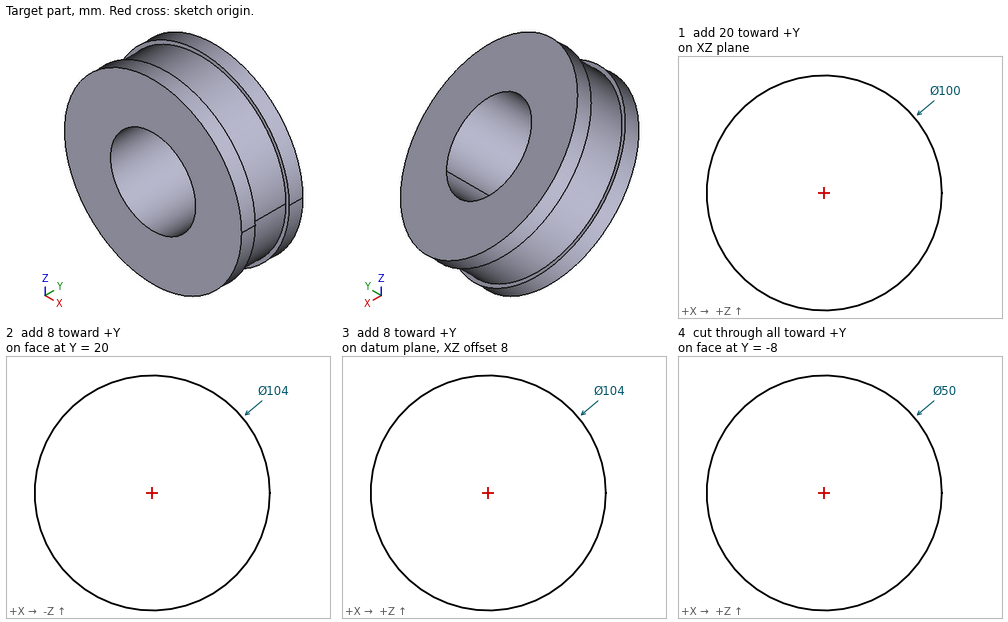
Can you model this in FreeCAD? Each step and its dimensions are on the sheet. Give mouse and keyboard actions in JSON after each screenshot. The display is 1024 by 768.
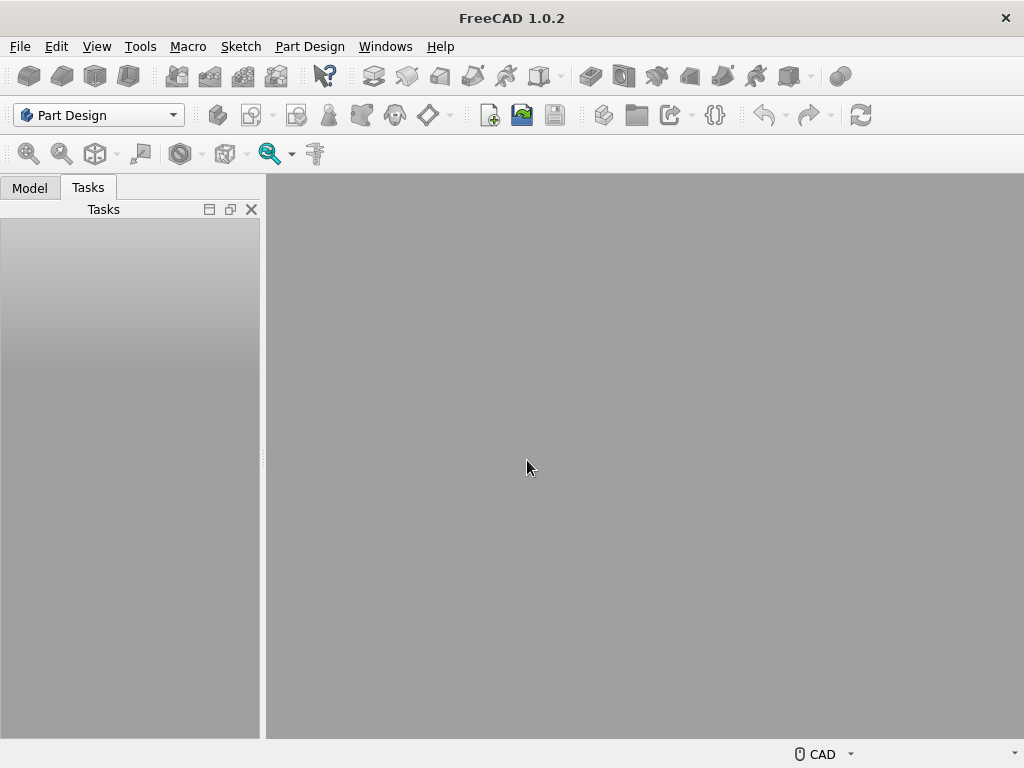
{"action": "key", "text": "ctrl+n"}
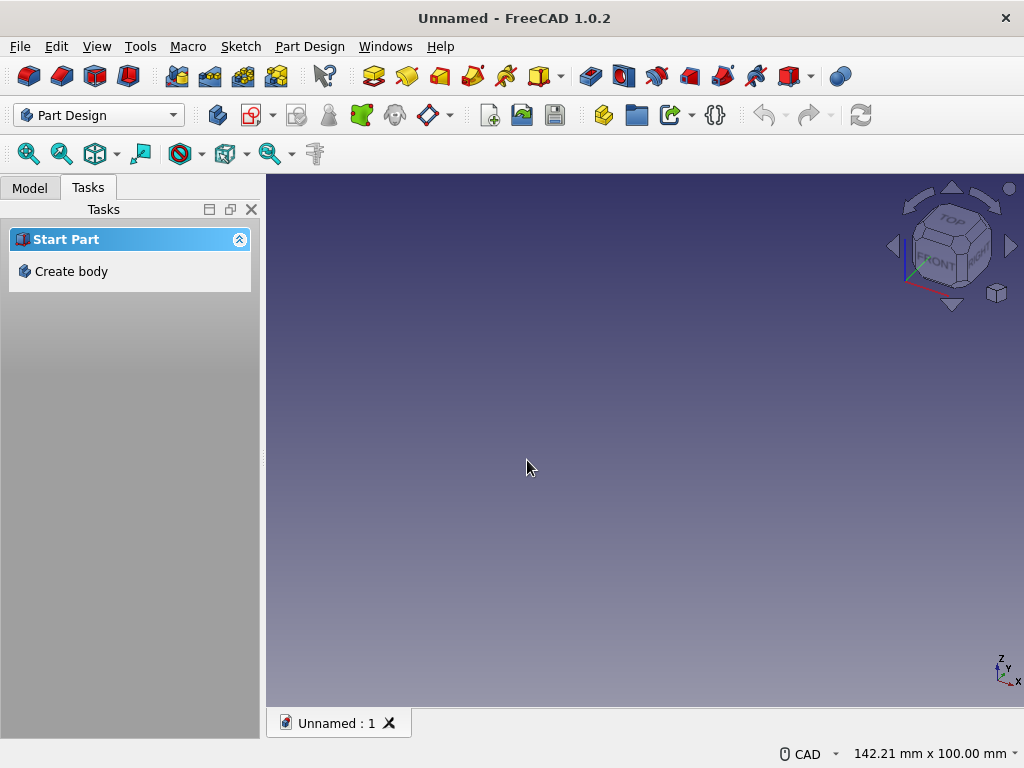
{"action": "left_click", "coordinate": [250, 116]}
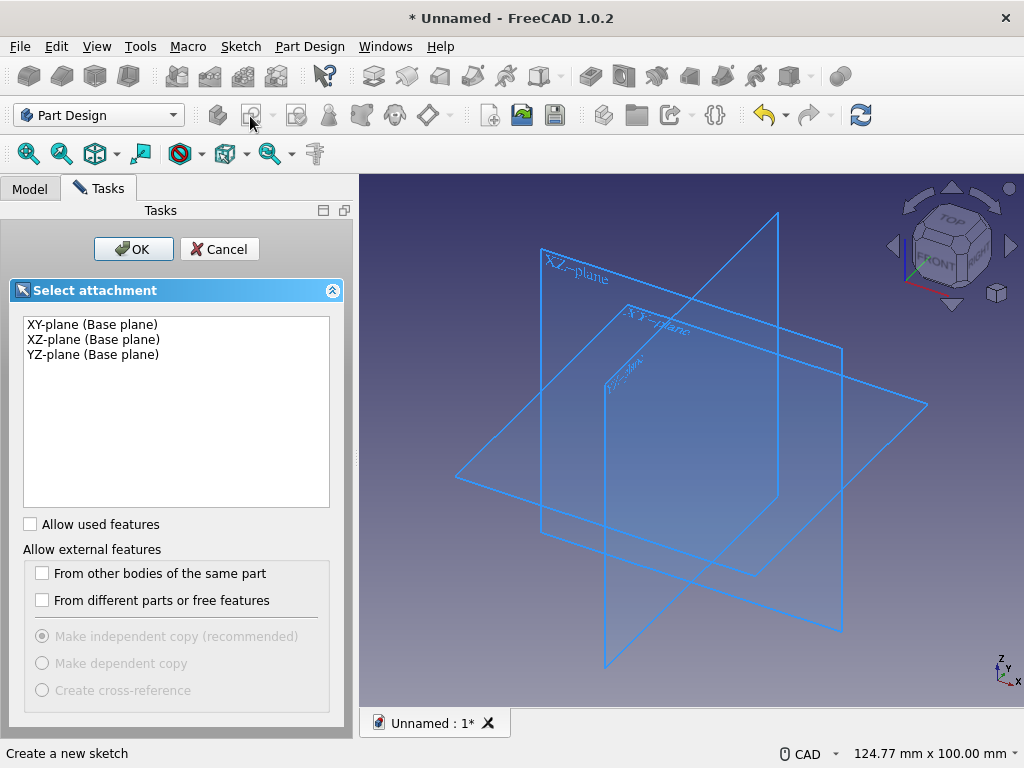
{"action": "left_click", "coordinate": [84, 340]}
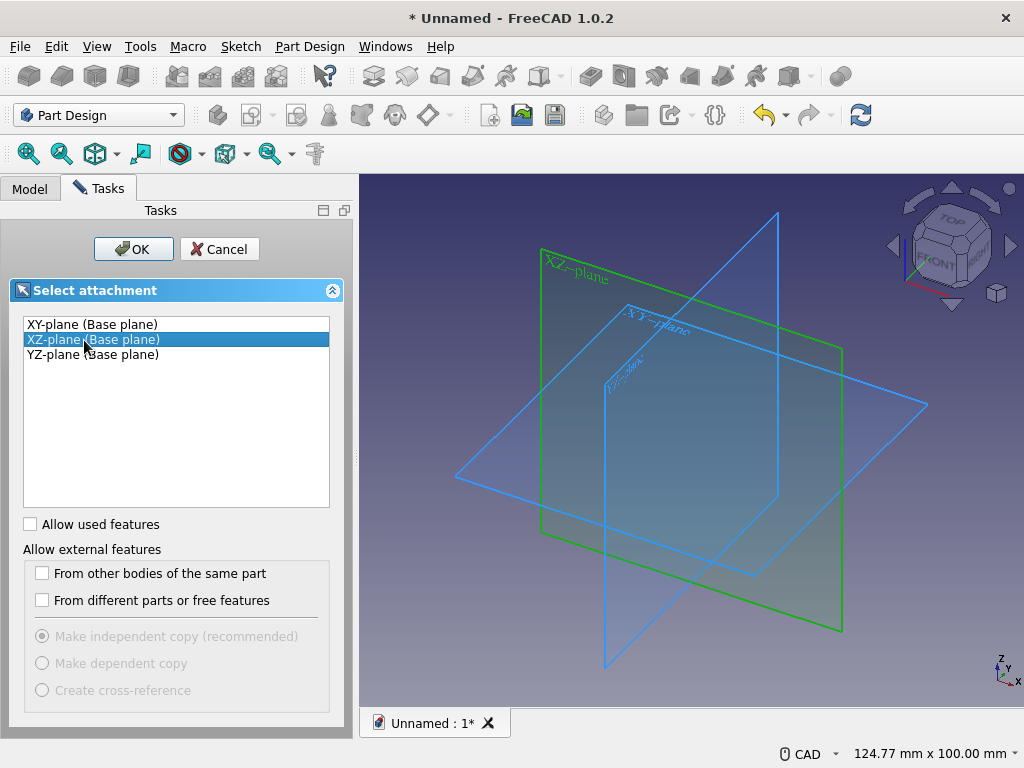
{"action": "left_click", "coordinate": [134, 249]}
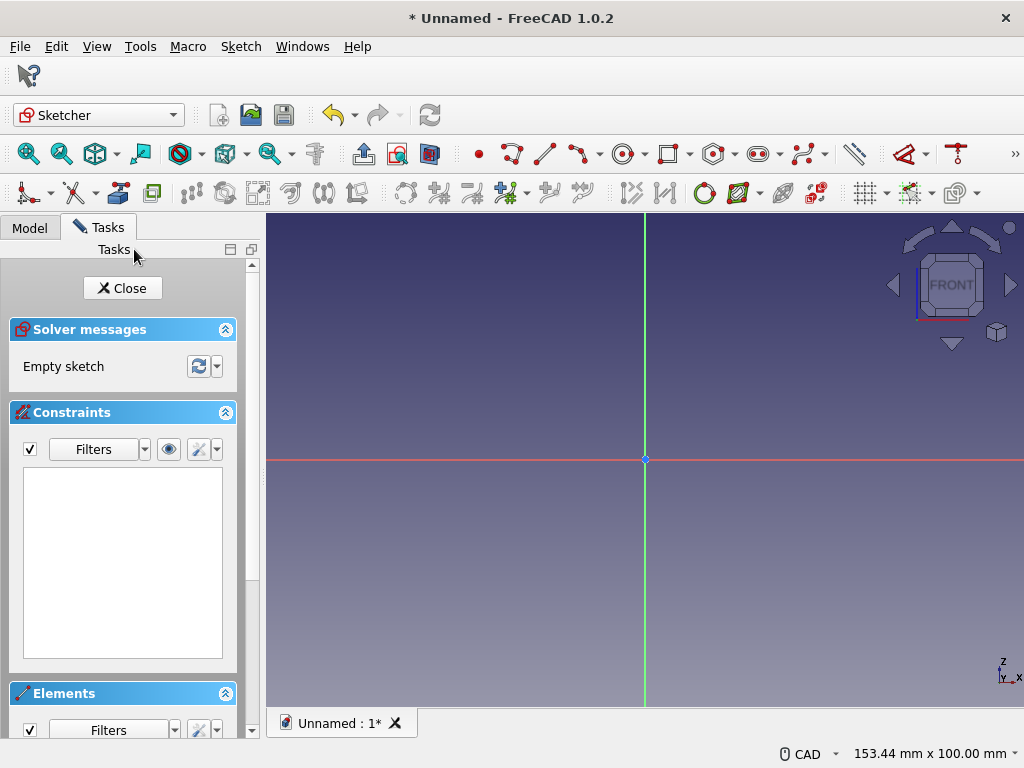
{"action": "scroll", "coordinate": [437, 460], "scroll_direction": "down", "scroll_amount": 2}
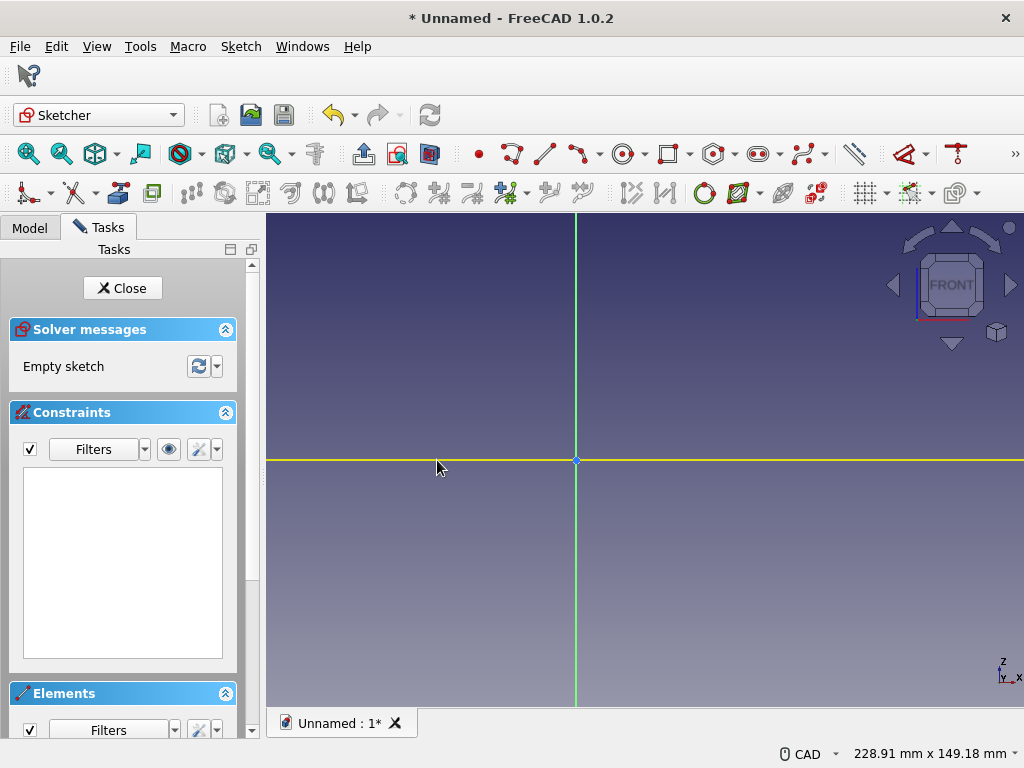
{"action": "left_click", "coordinate": [622, 154]}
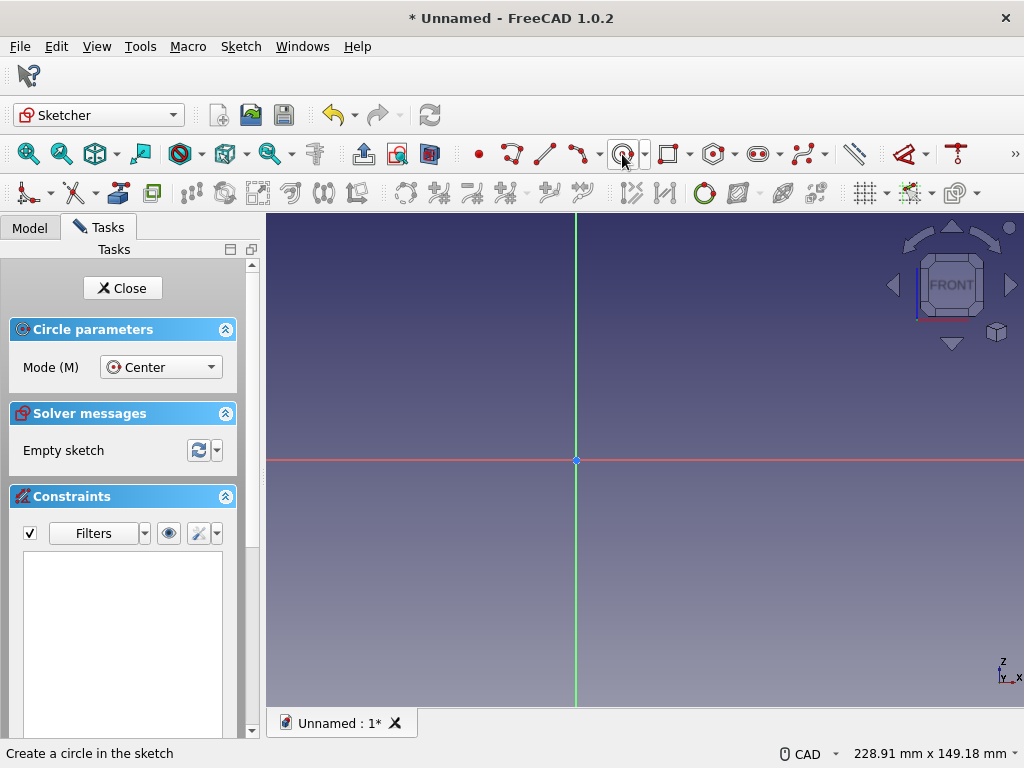
{"action": "left_click", "coordinate": [577, 460]}
{"action": "mouse_move", "coordinate": [694, 343]}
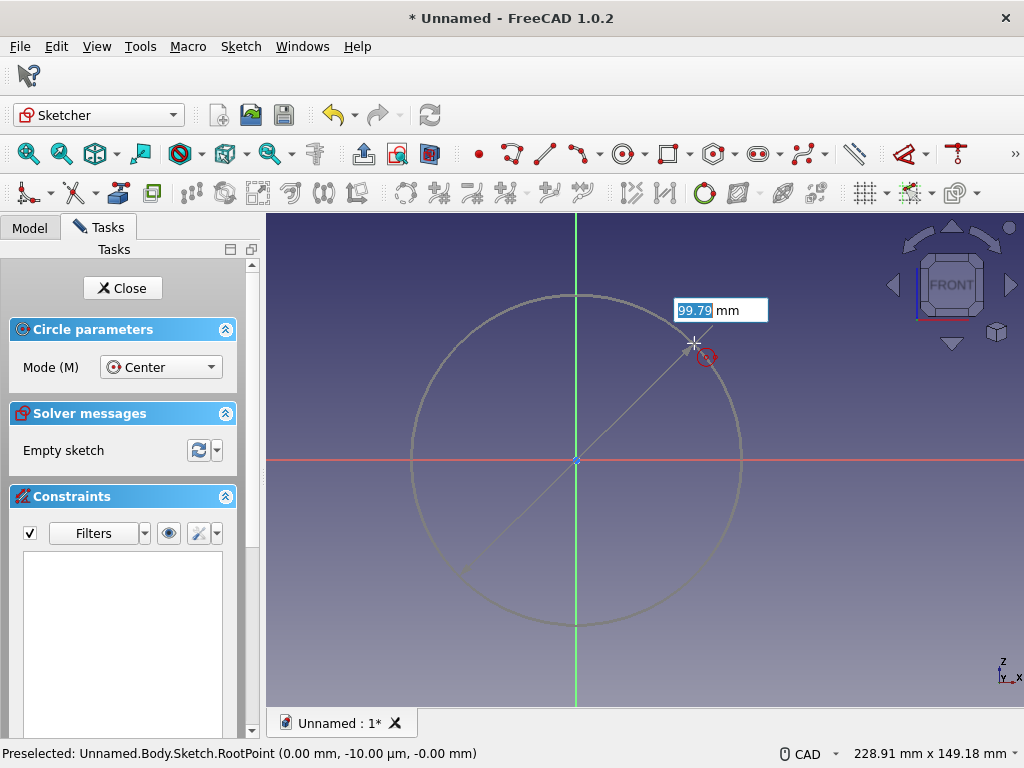
{"action": "type", "text": "100"}
{"action": "key", "text": "Return"}
{"action": "key", "text": "Escape"}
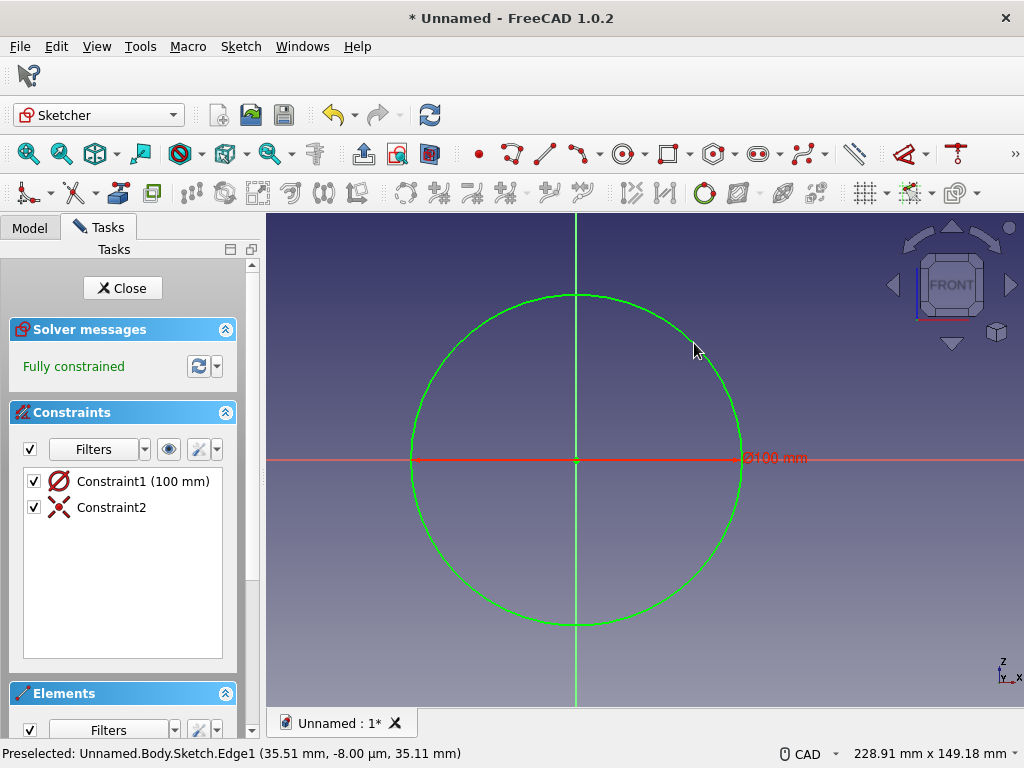
{"action": "left_click", "coordinate": [123, 288]}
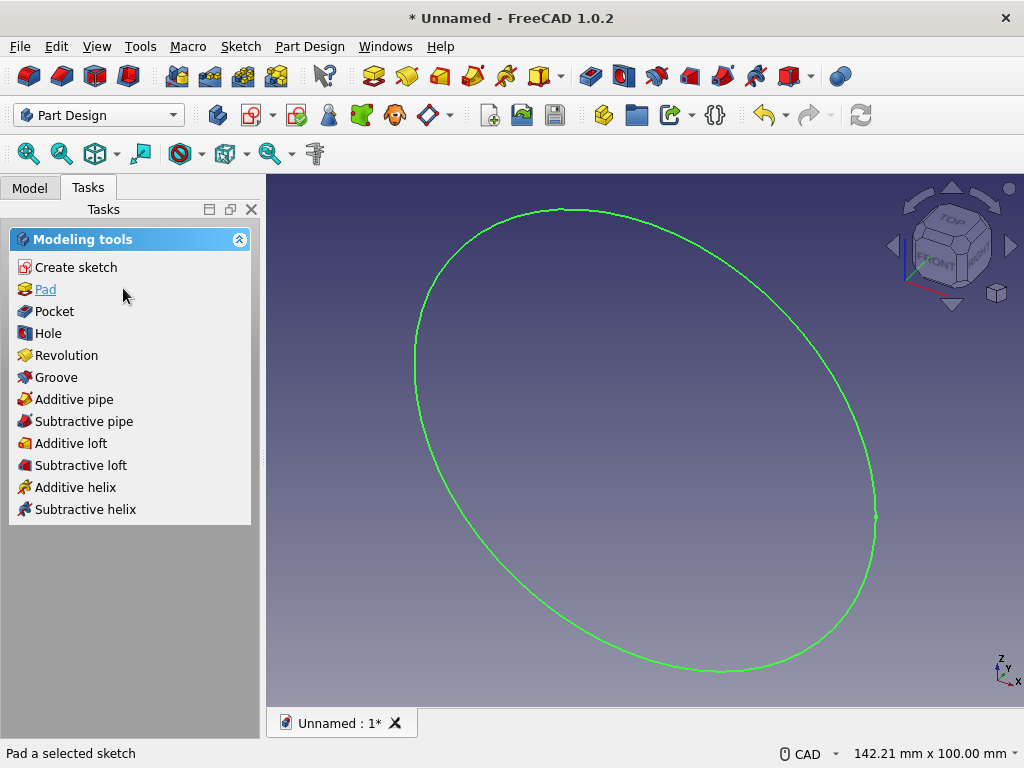
{"action": "left_click", "coordinate": [374, 76]}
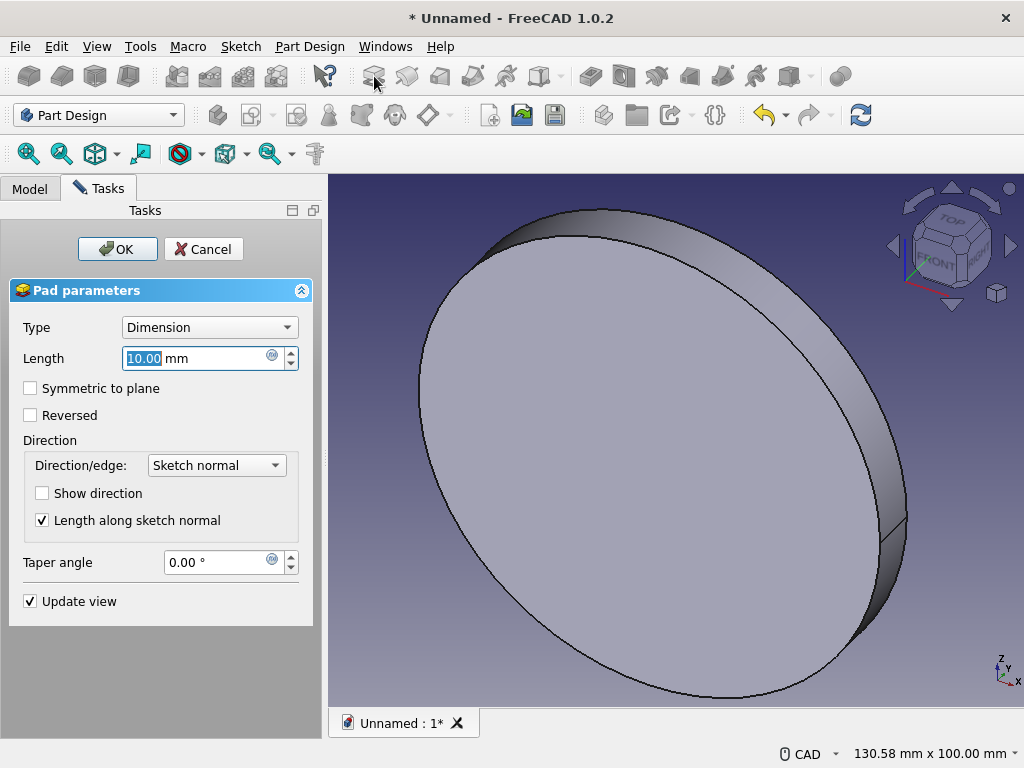
{"action": "type", "text": "20"}
{"action": "key", "text": "Tab"}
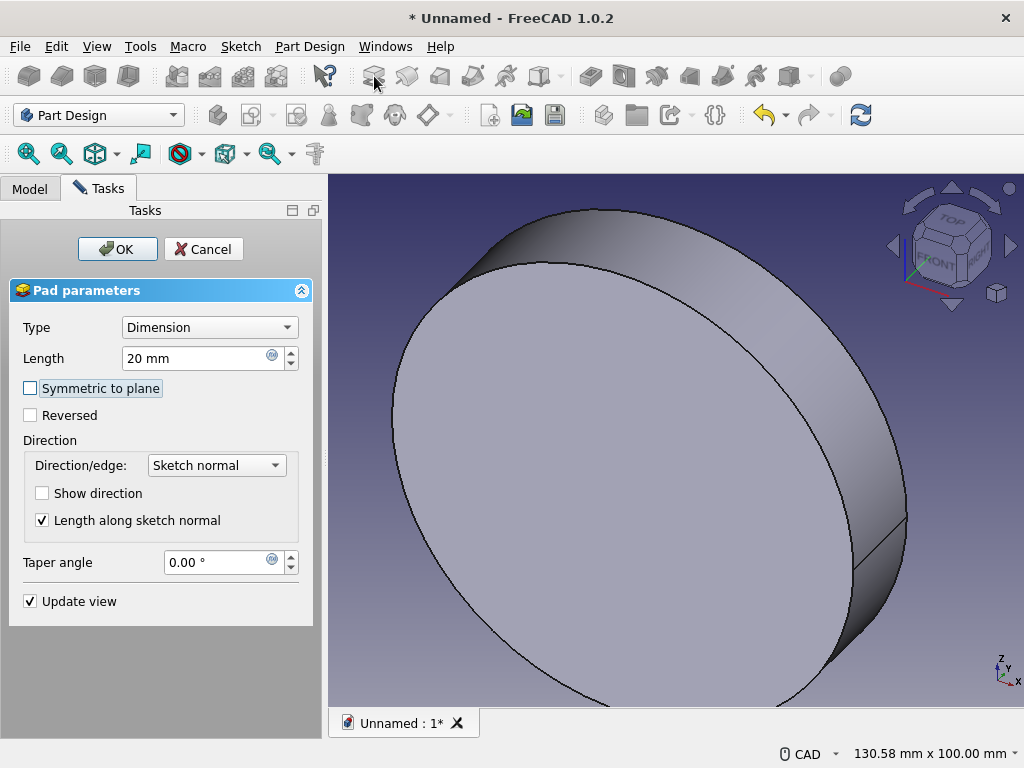
{"action": "left_click", "coordinate": [31, 415]}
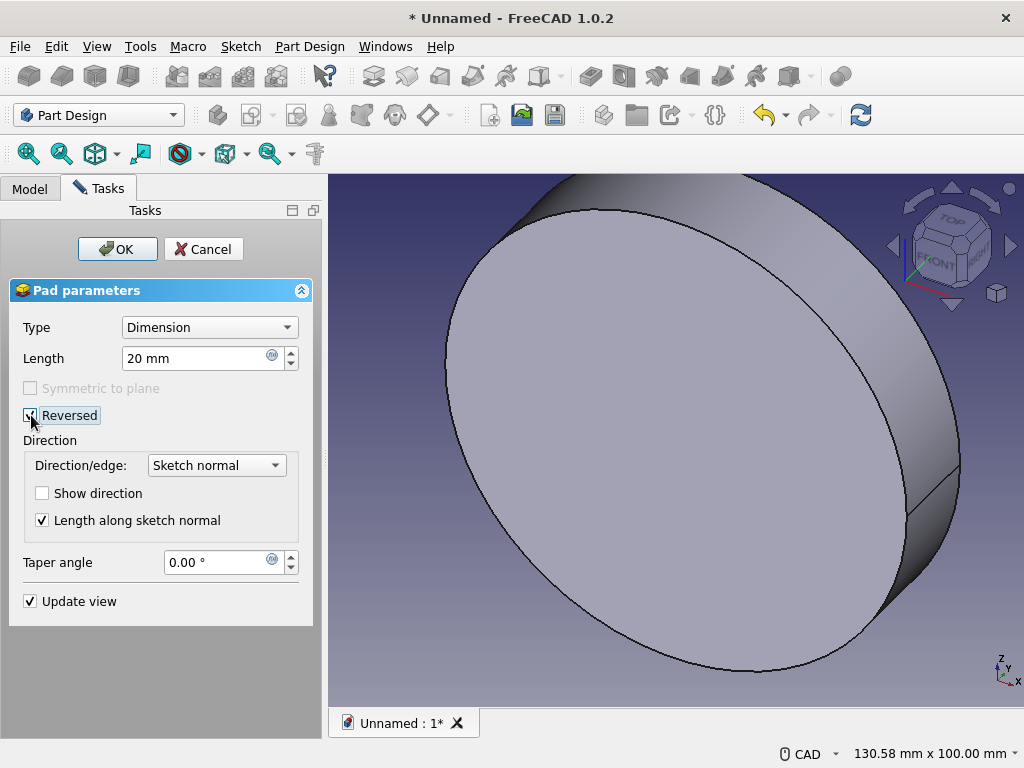
{"action": "left_click", "coordinate": [118, 249]}